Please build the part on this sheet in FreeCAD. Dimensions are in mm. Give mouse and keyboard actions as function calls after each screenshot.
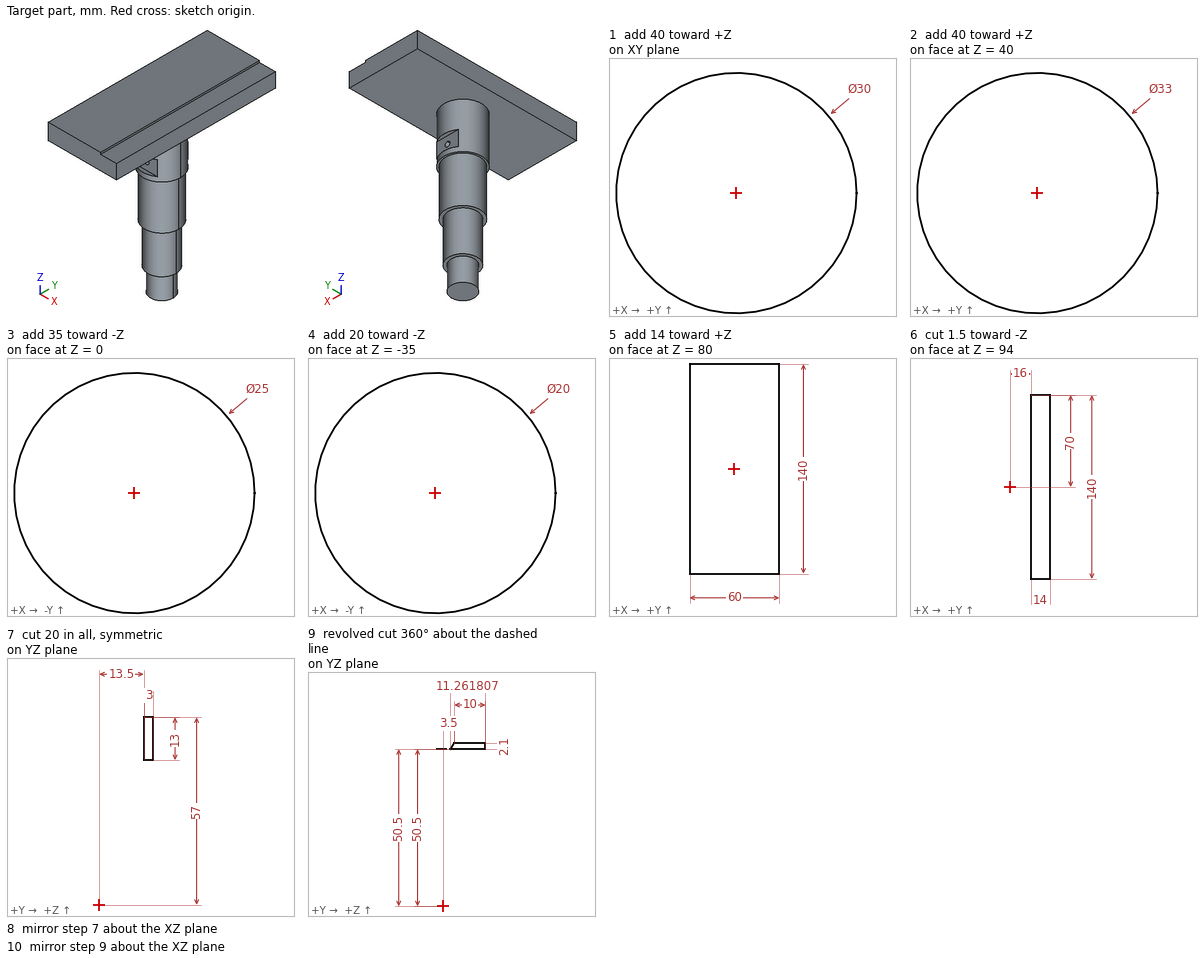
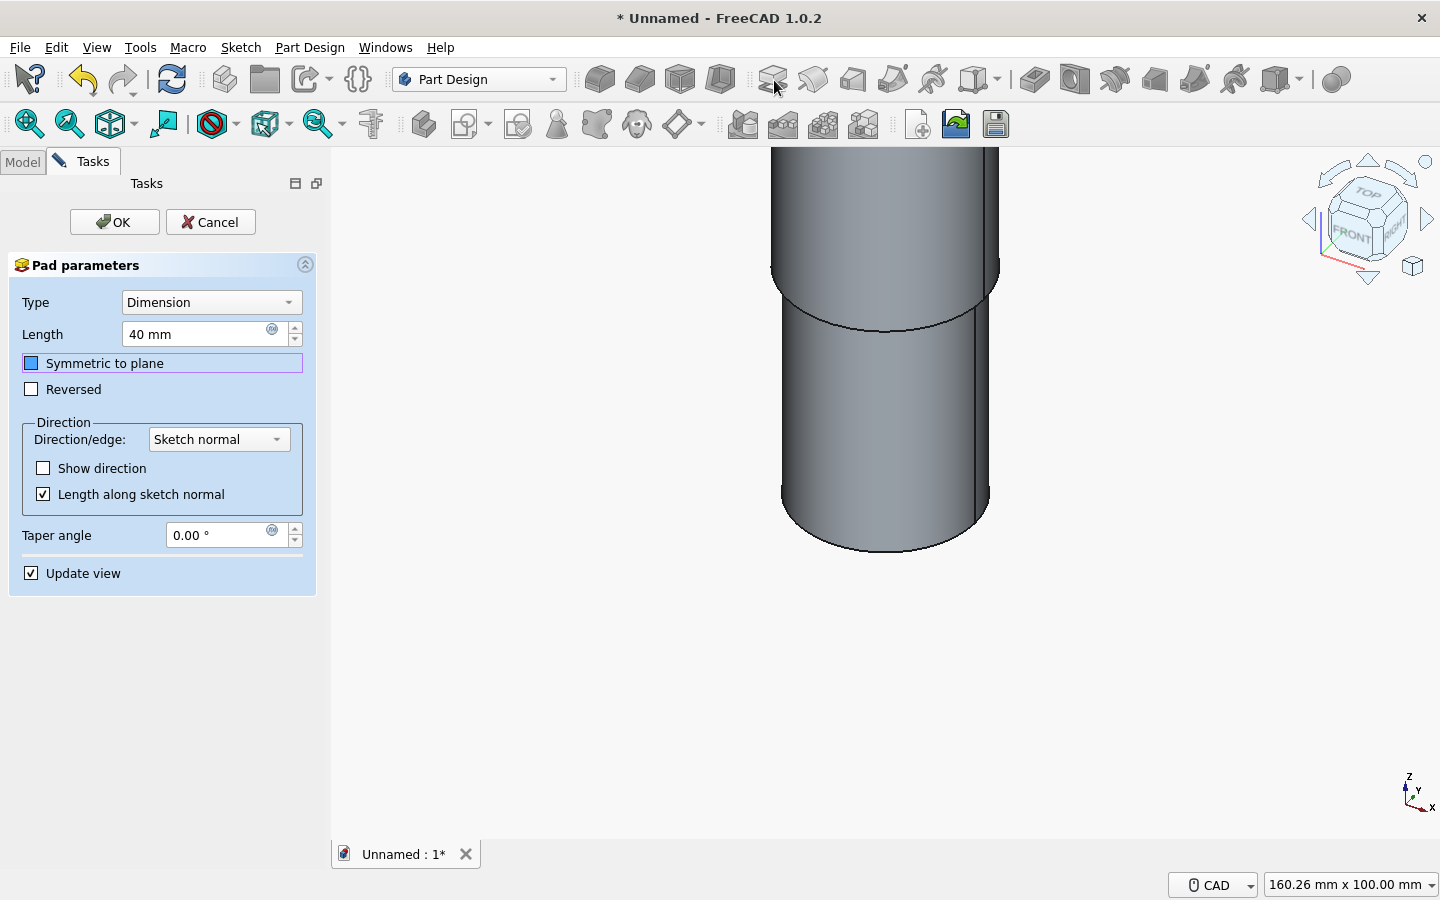
click(115, 222)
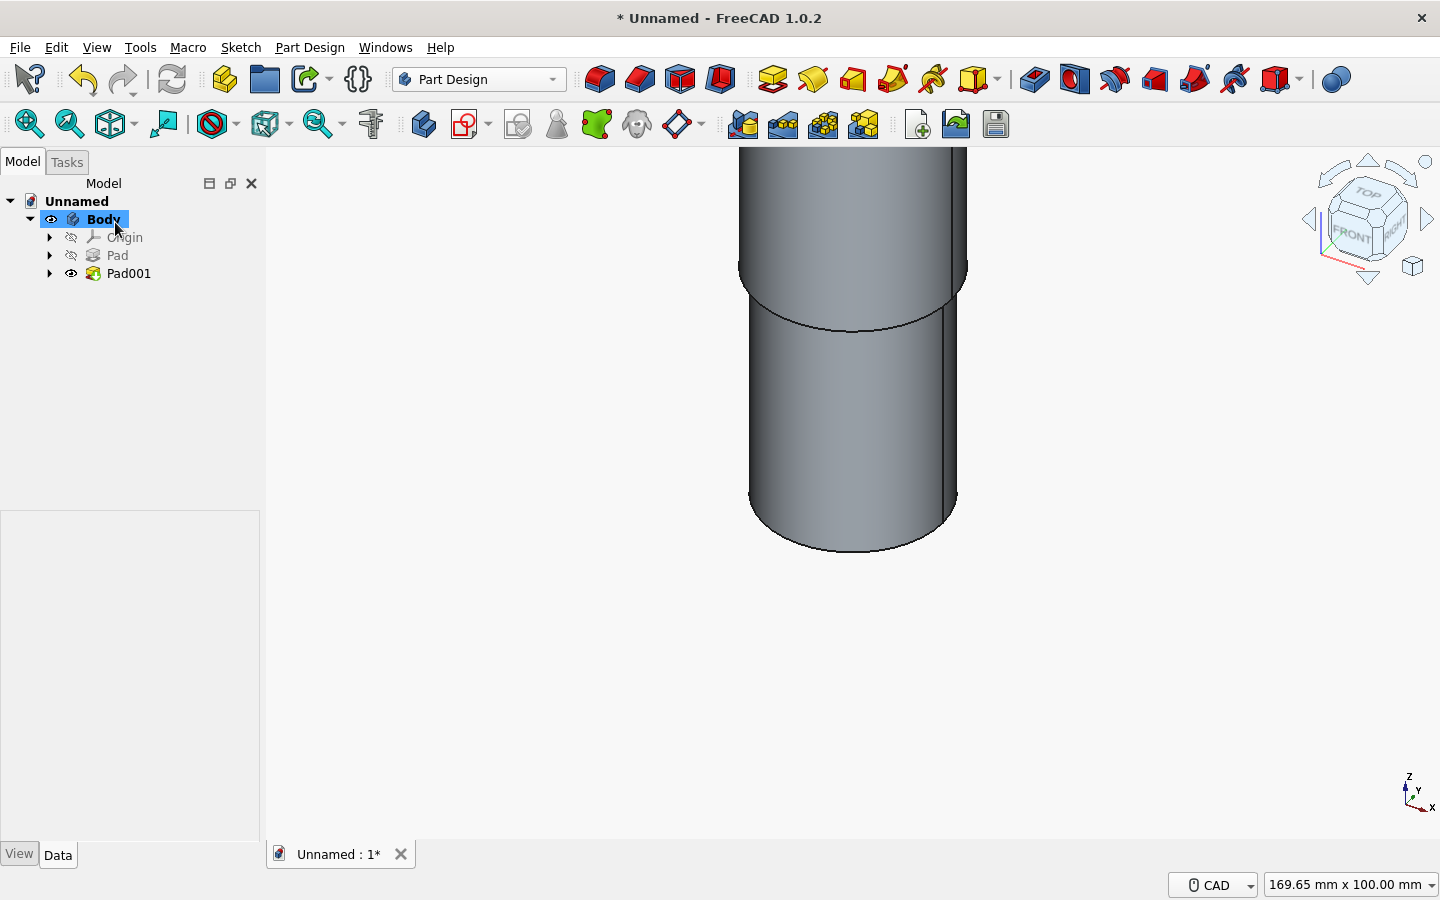
click(30, 124)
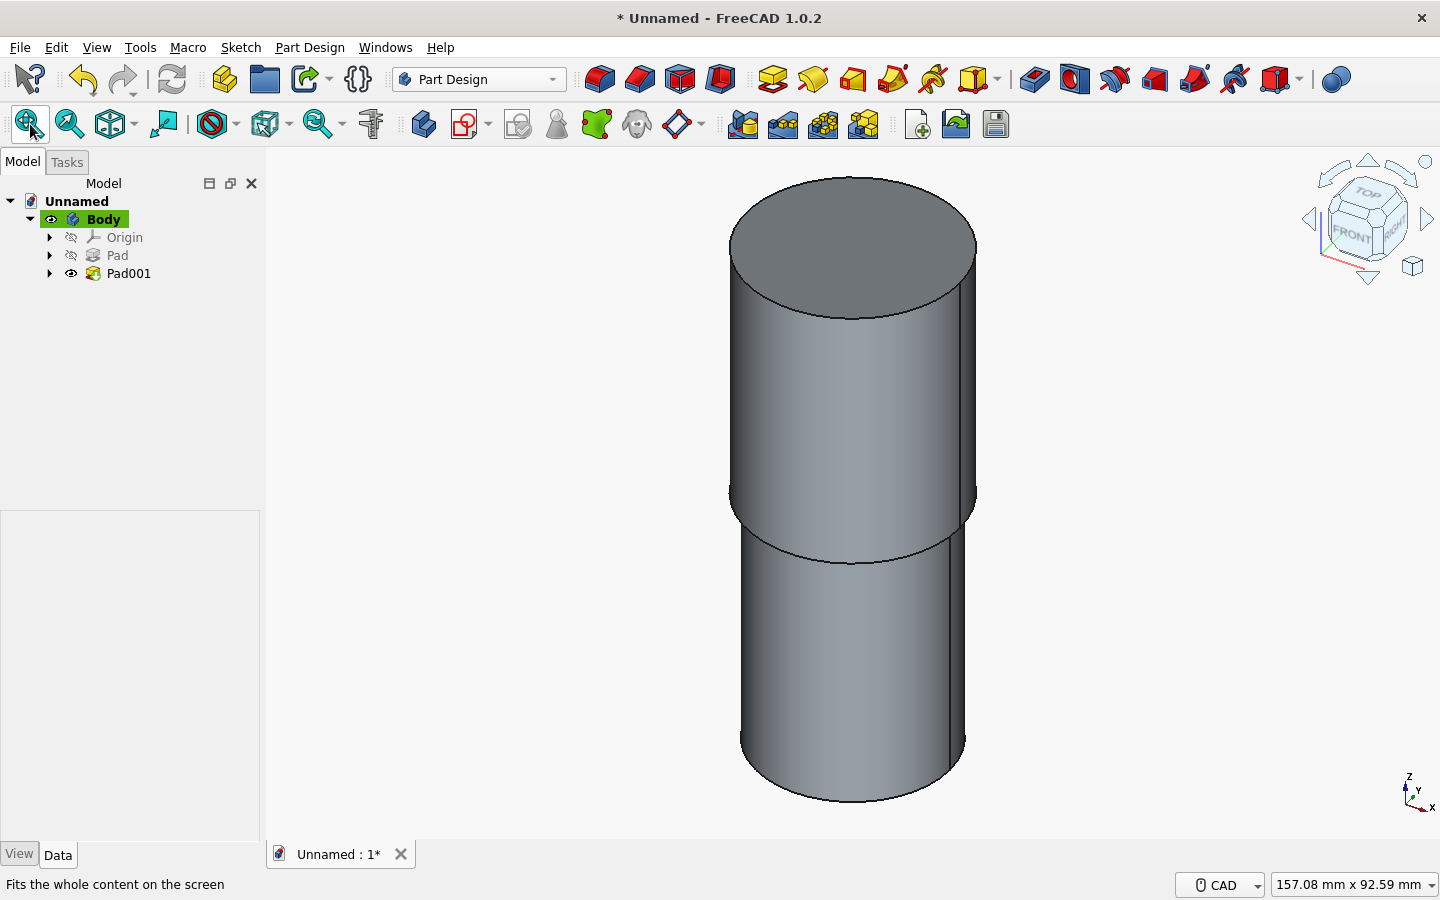
key(5)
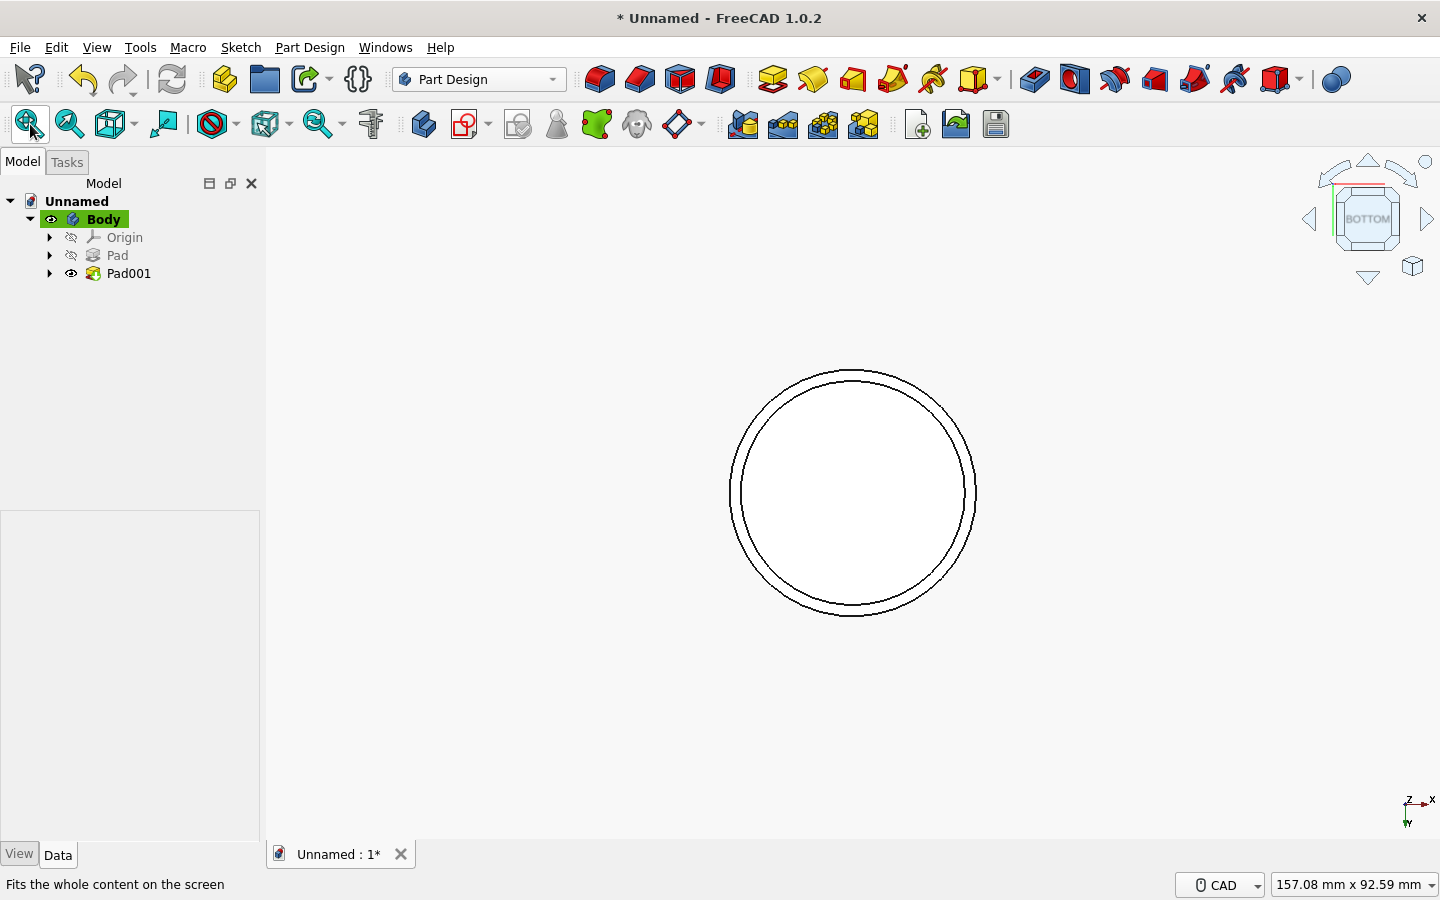
click(30, 124)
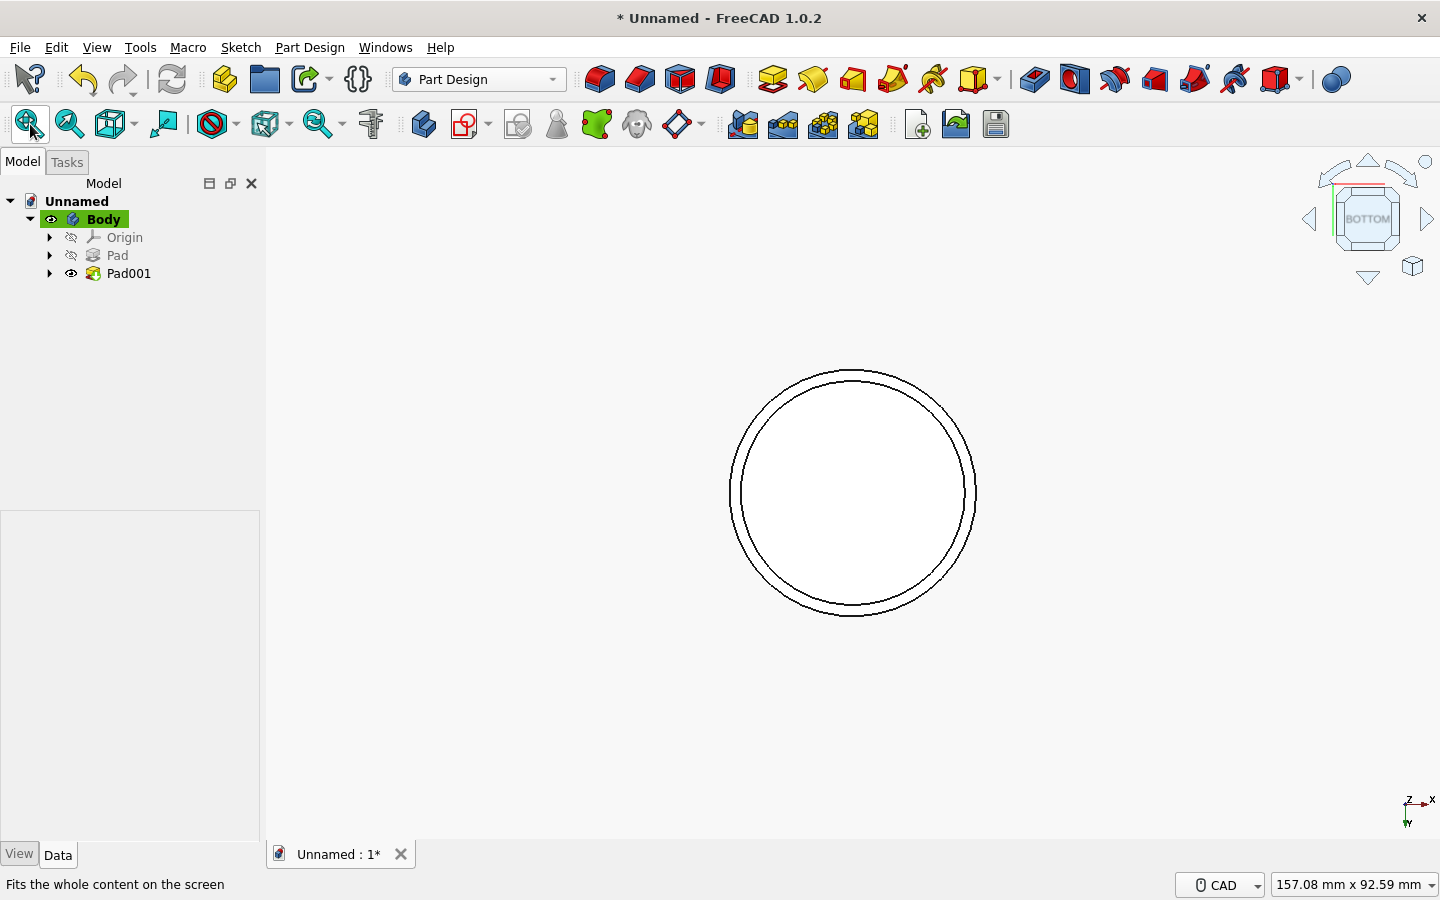
click(853, 492)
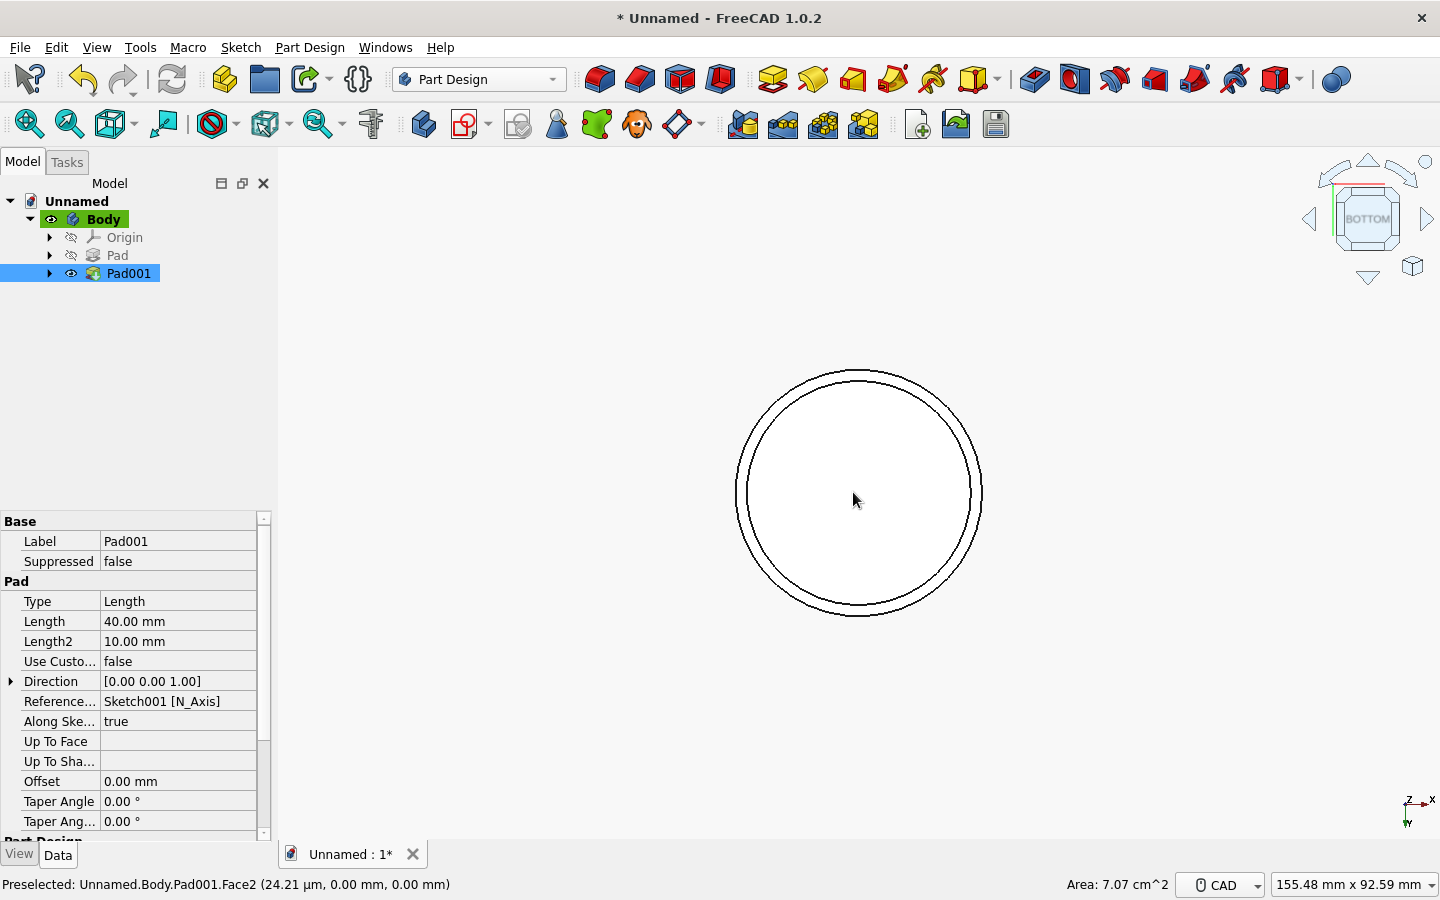
click(464, 124)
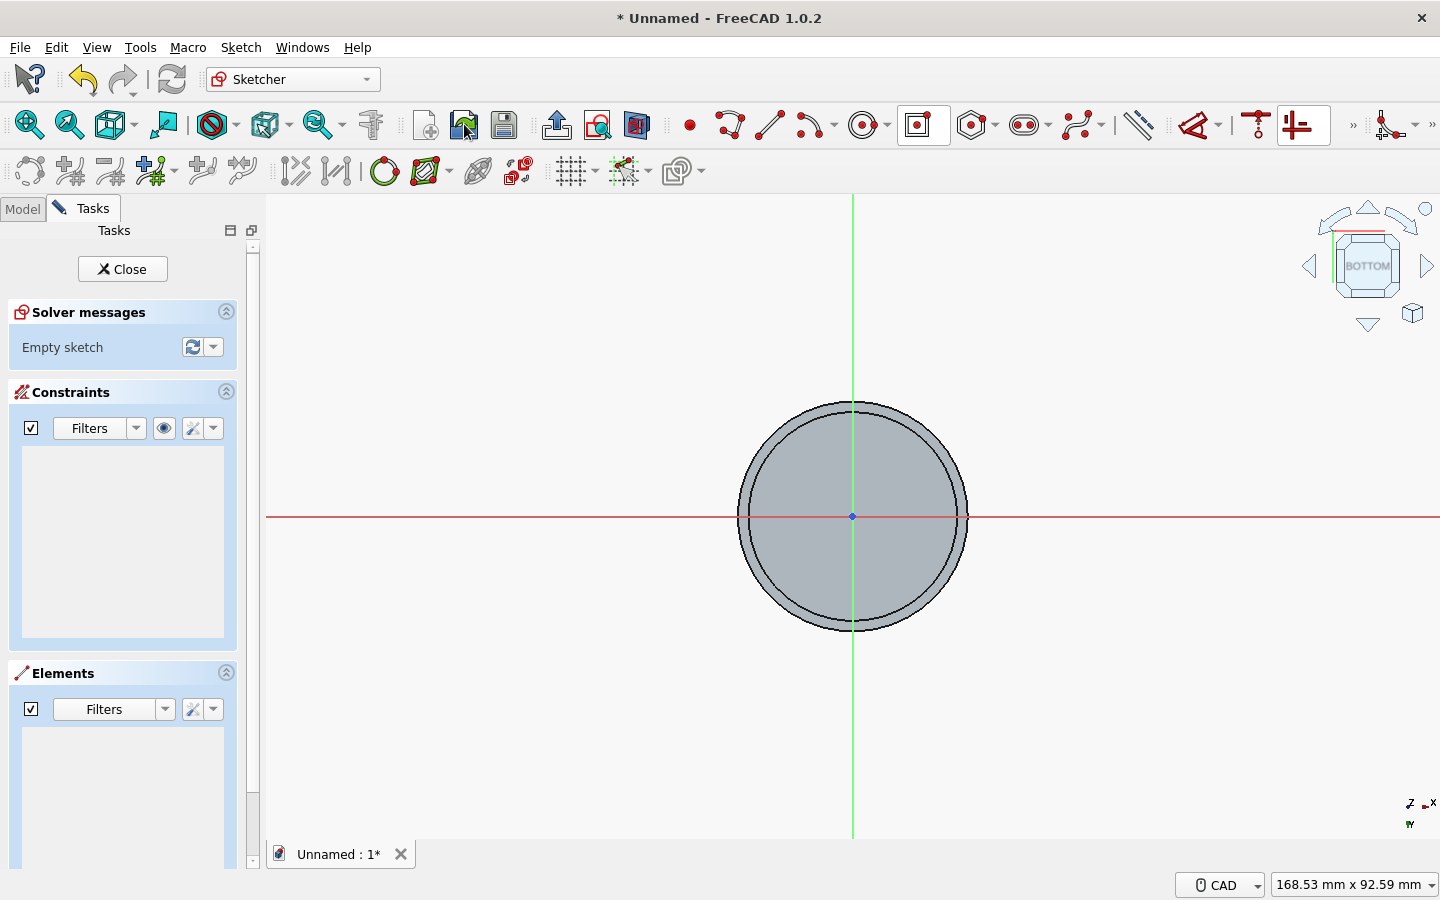
scroll(909, 517, up, 4)